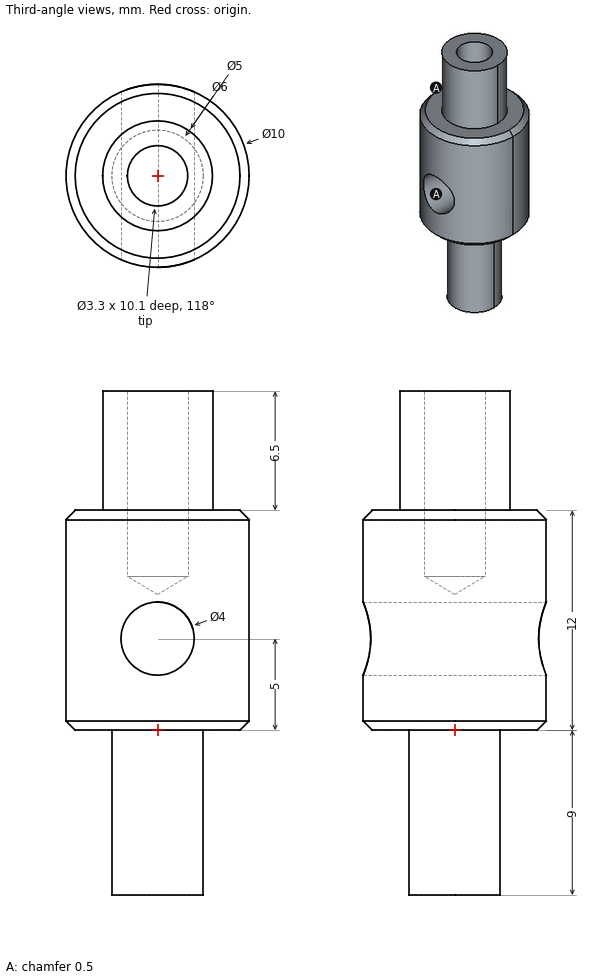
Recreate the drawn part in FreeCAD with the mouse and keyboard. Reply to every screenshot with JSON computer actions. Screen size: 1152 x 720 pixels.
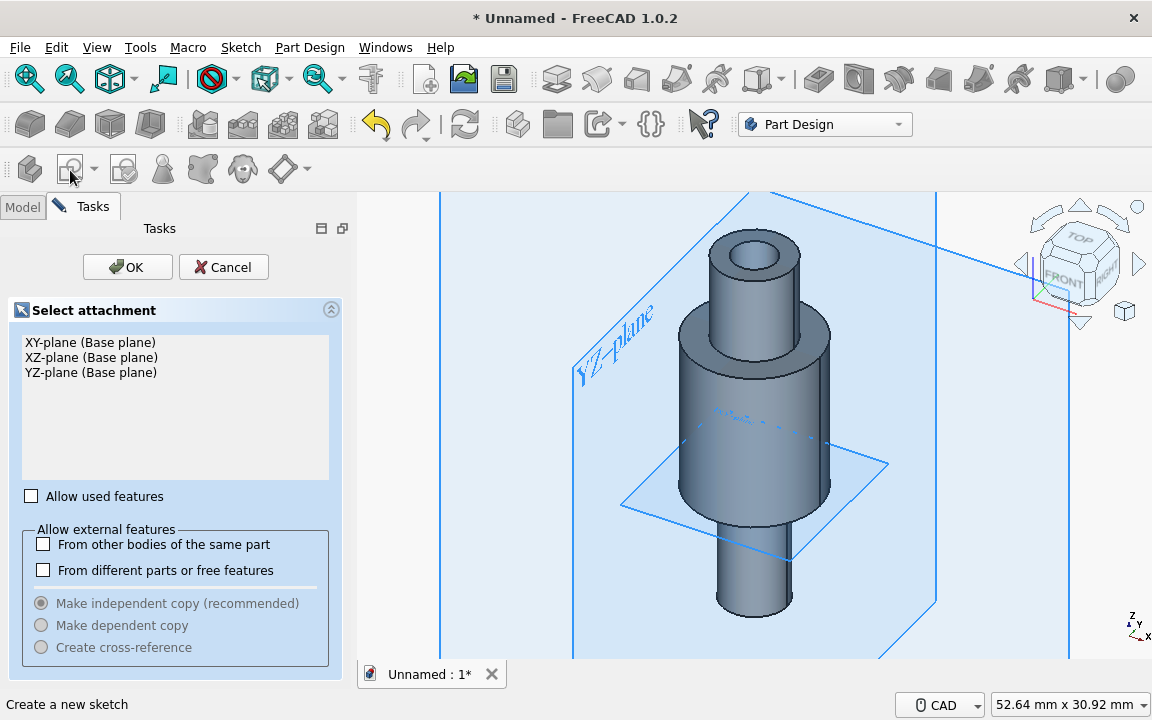
{"action": "left_click", "coordinate": [82, 358]}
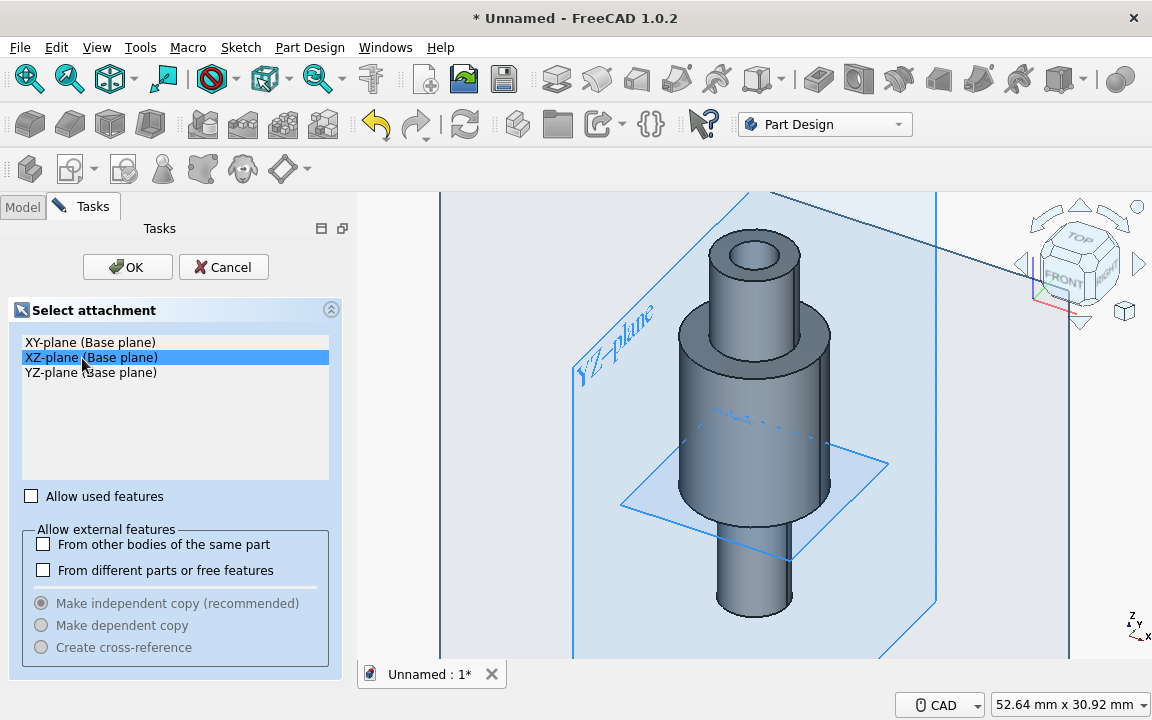
{"action": "left_click", "coordinate": [128, 267]}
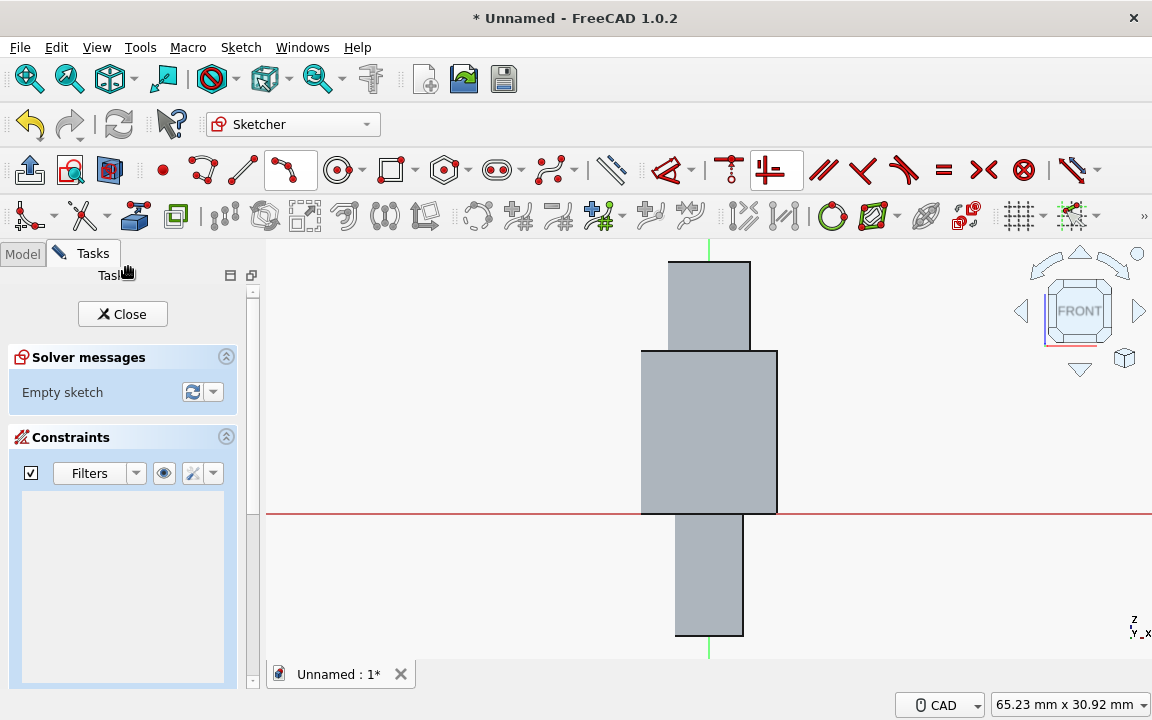
{"action": "key", "text": "q s"}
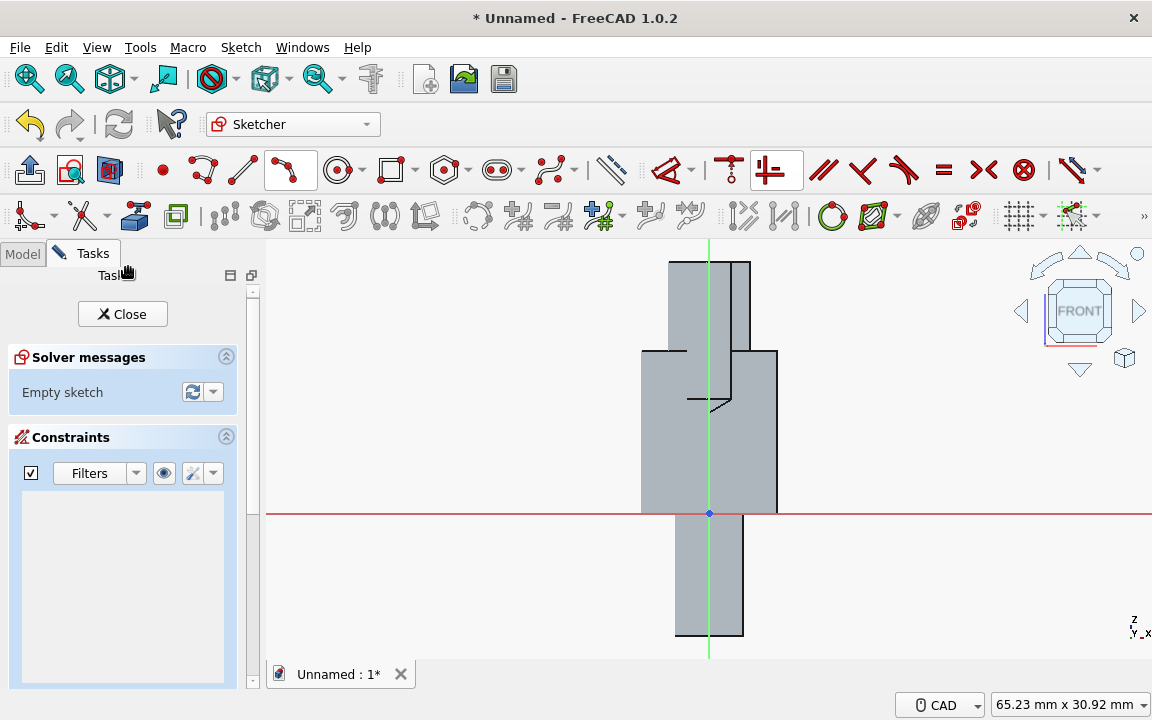
{"action": "scroll", "coordinate": [749, 476], "scroll_direction": "up", "scroll_amount": 5}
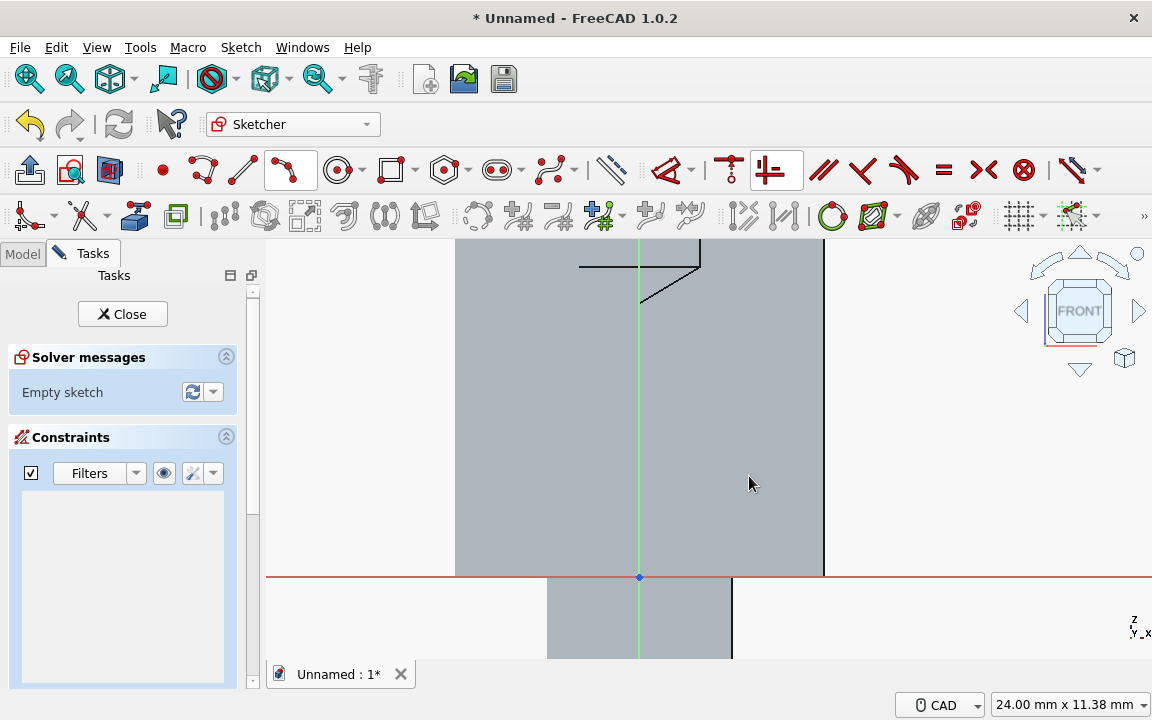
{"action": "key", "text": "g c"}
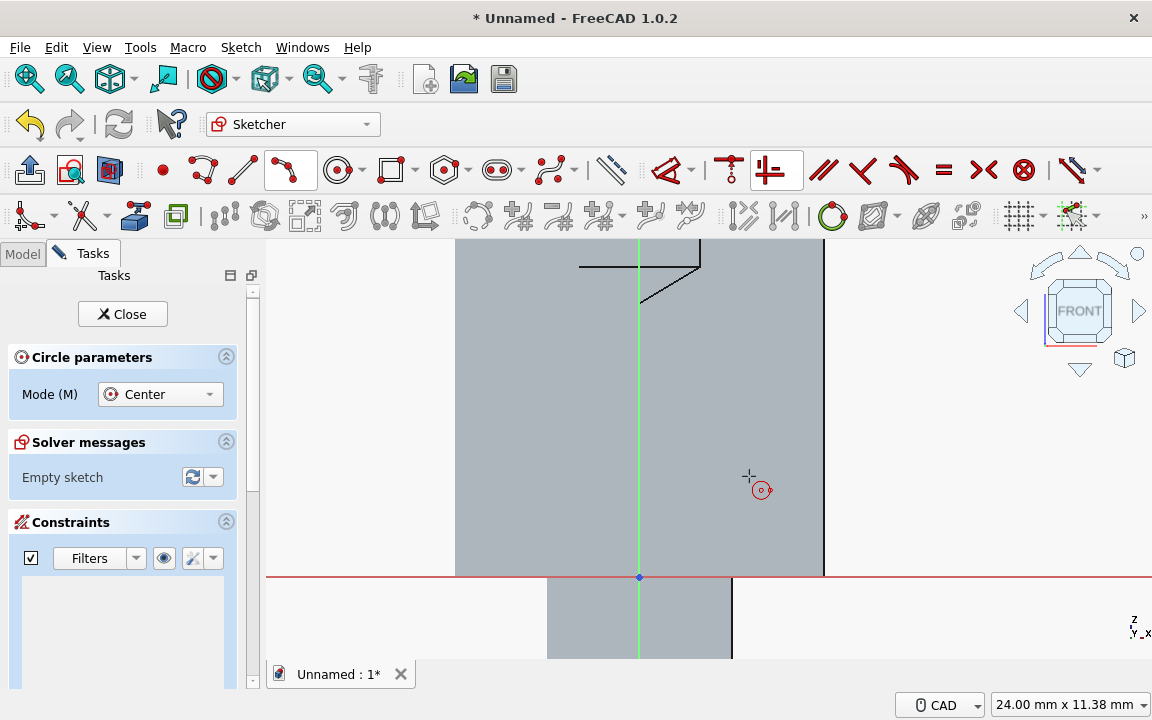
{"action": "left_click", "coordinate": [639, 392]}
{"action": "left_click", "coordinate": [692, 340]}
{"action": "key", "text": "Escape"}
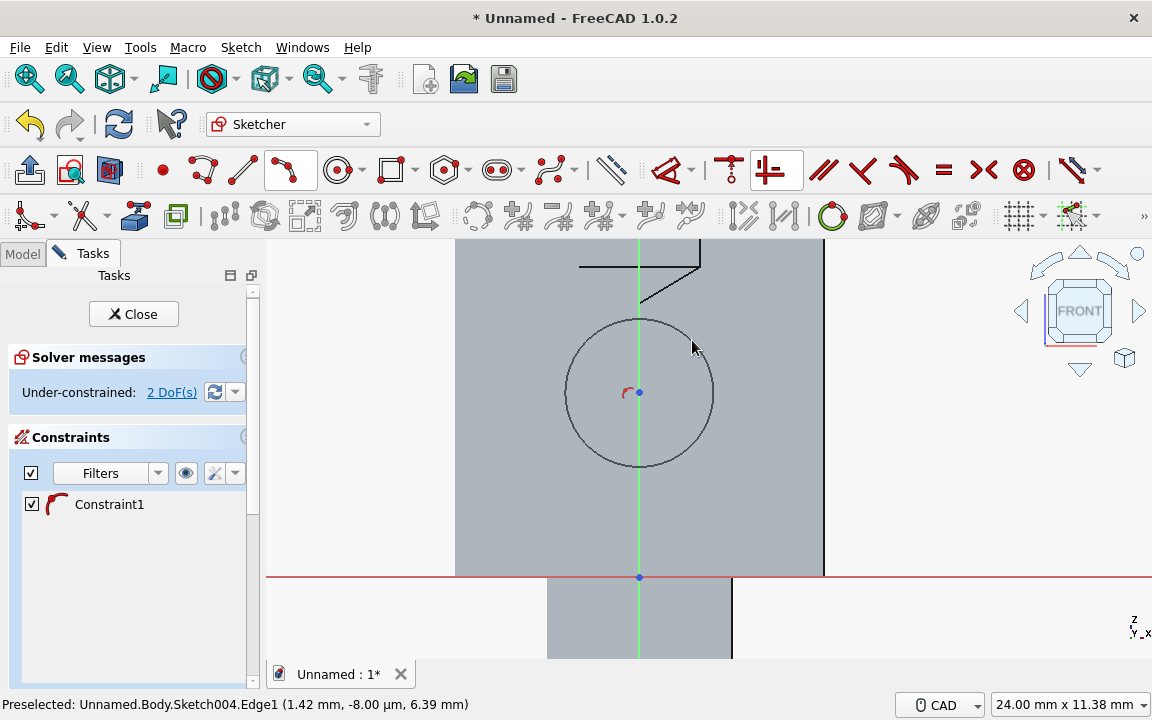
{"action": "left_click", "coordinate": [666, 170]}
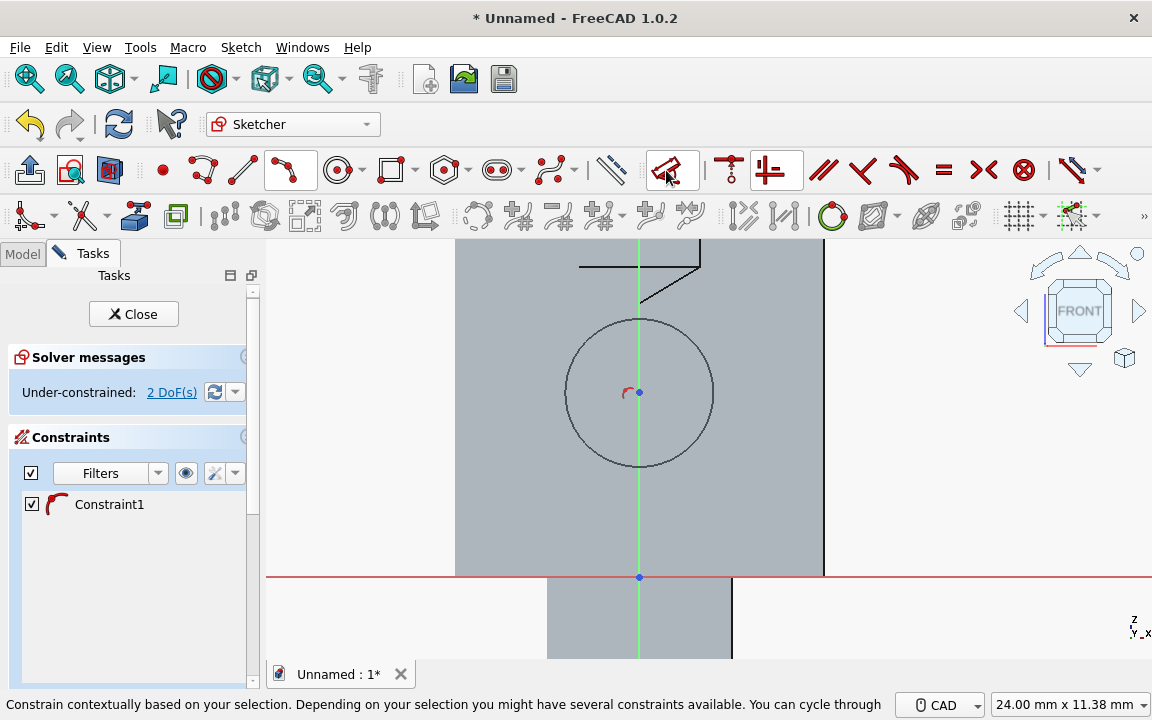
{"action": "left_click", "coordinate": [692, 341]}
{"action": "left_click", "coordinate": [715, 319]}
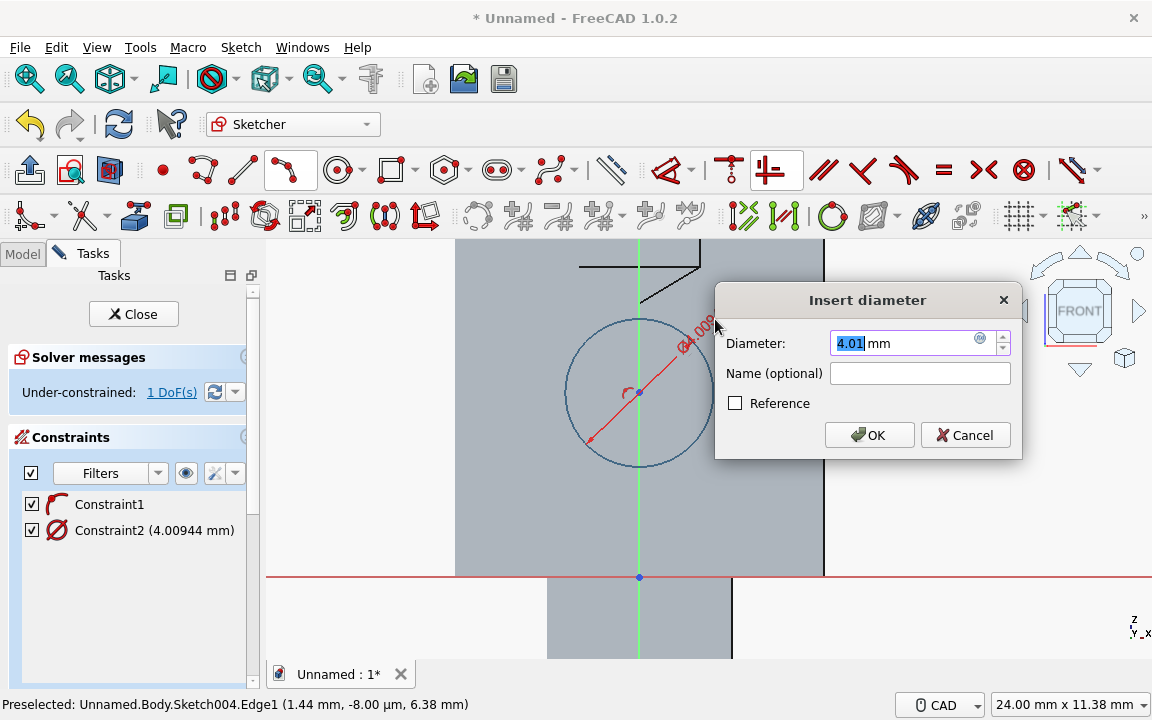
{"action": "type", "text": "4"}
{"action": "key", "text": "Return"}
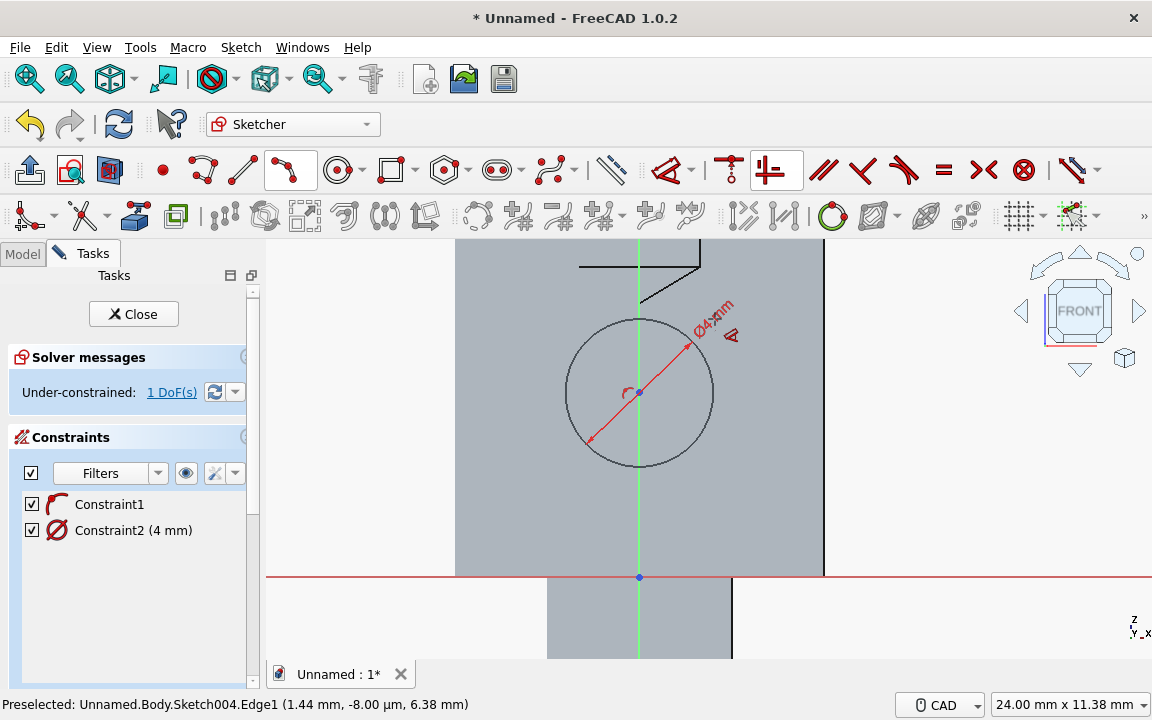
{"action": "left_click", "coordinate": [639, 393]}
{"action": "left_click", "coordinate": [673, 485]}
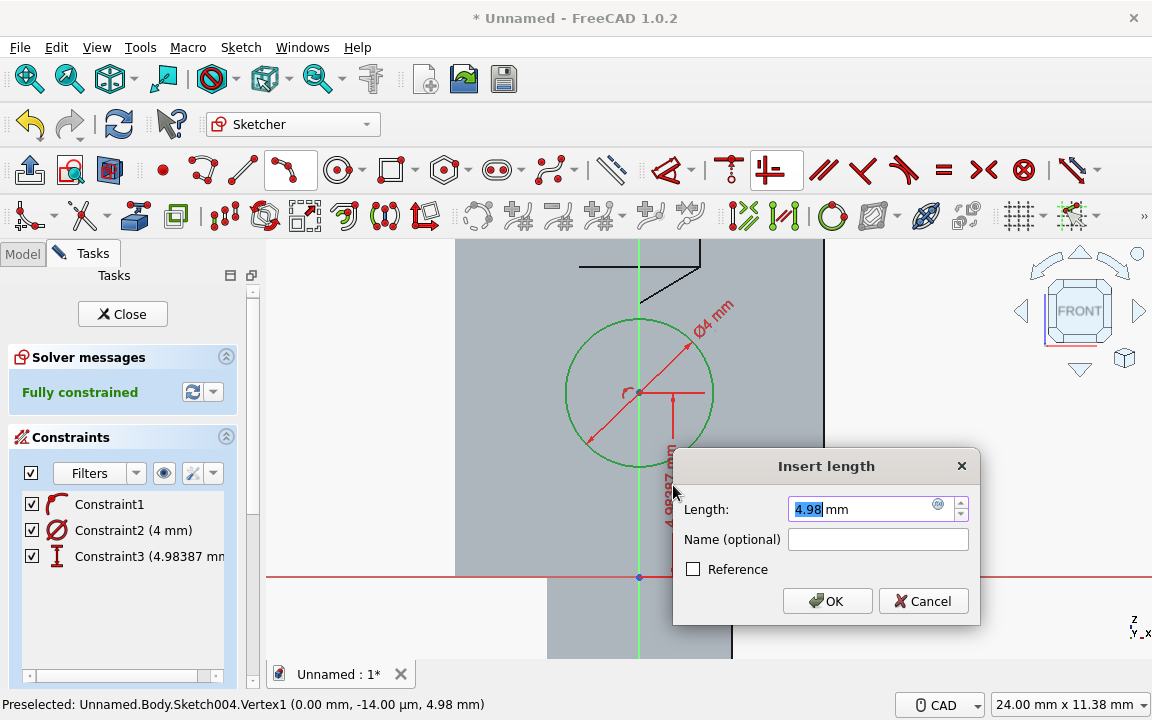
{"action": "type", "text": "5"}
{"action": "key", "text": "Return"}
{"action": "key", "text": "Escape"}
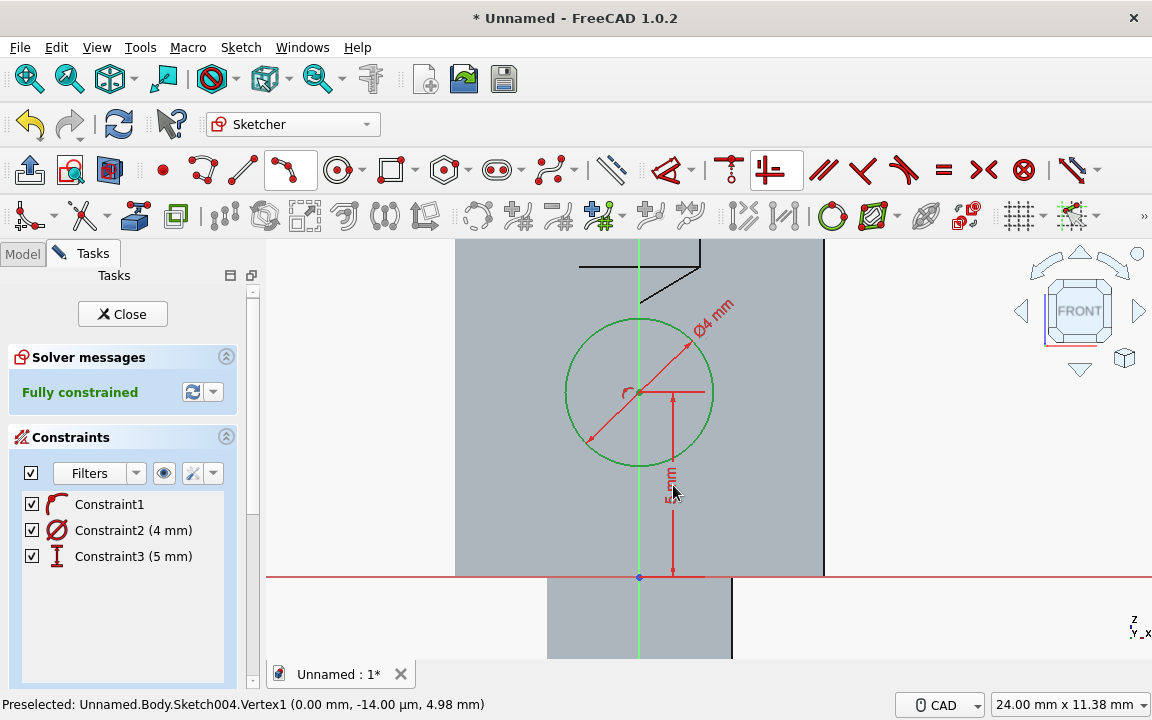
{"action": "left_click", "coordinate": [123, 314]}